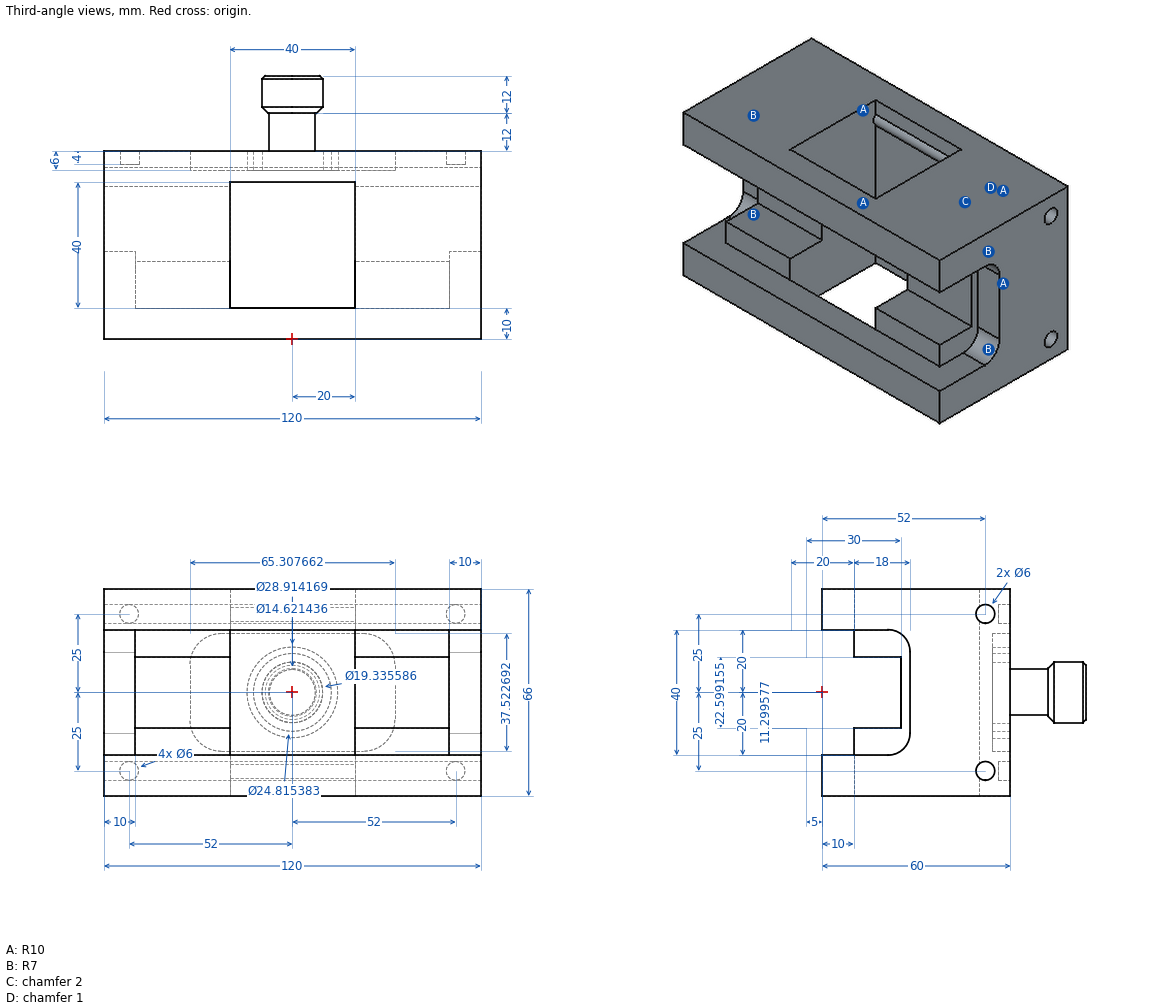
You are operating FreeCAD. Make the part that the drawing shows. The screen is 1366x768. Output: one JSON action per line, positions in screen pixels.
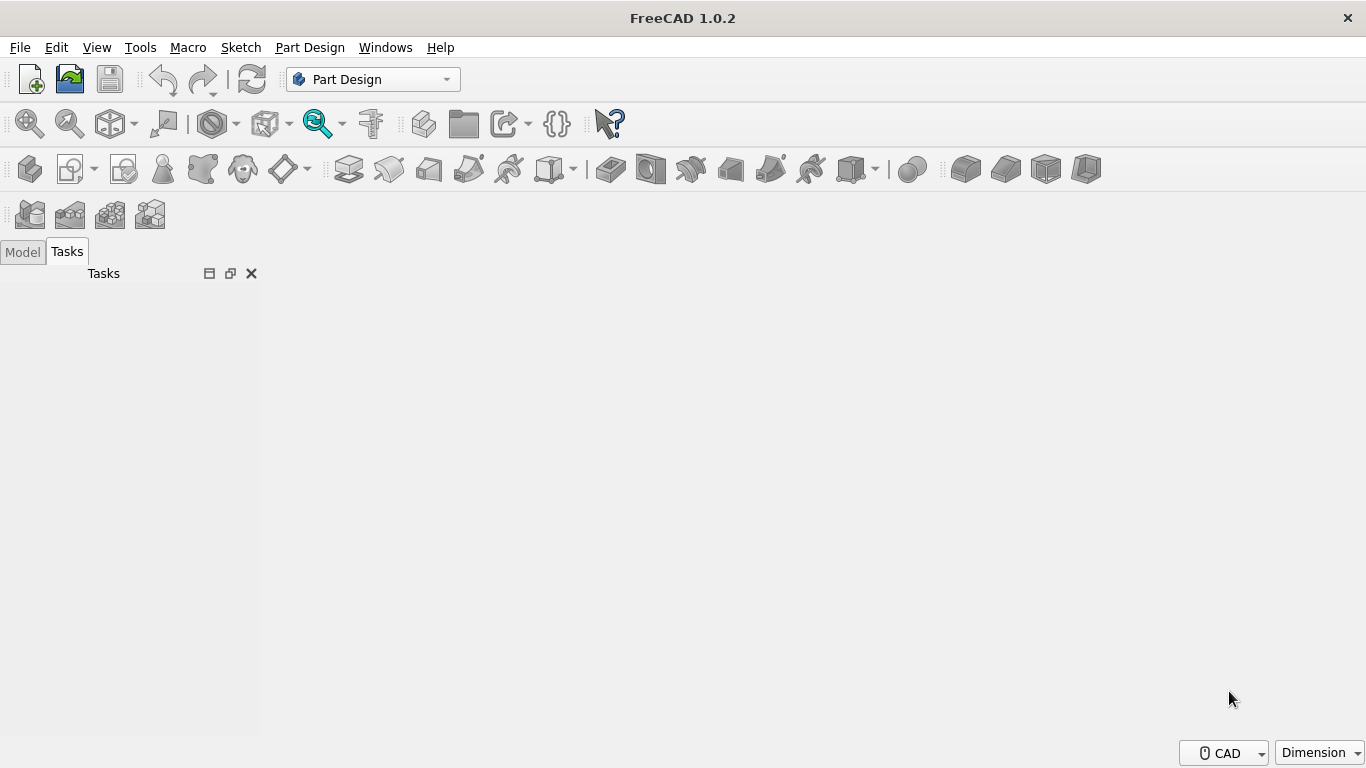
{"action": "left_click", "coordinate": [30, 80]}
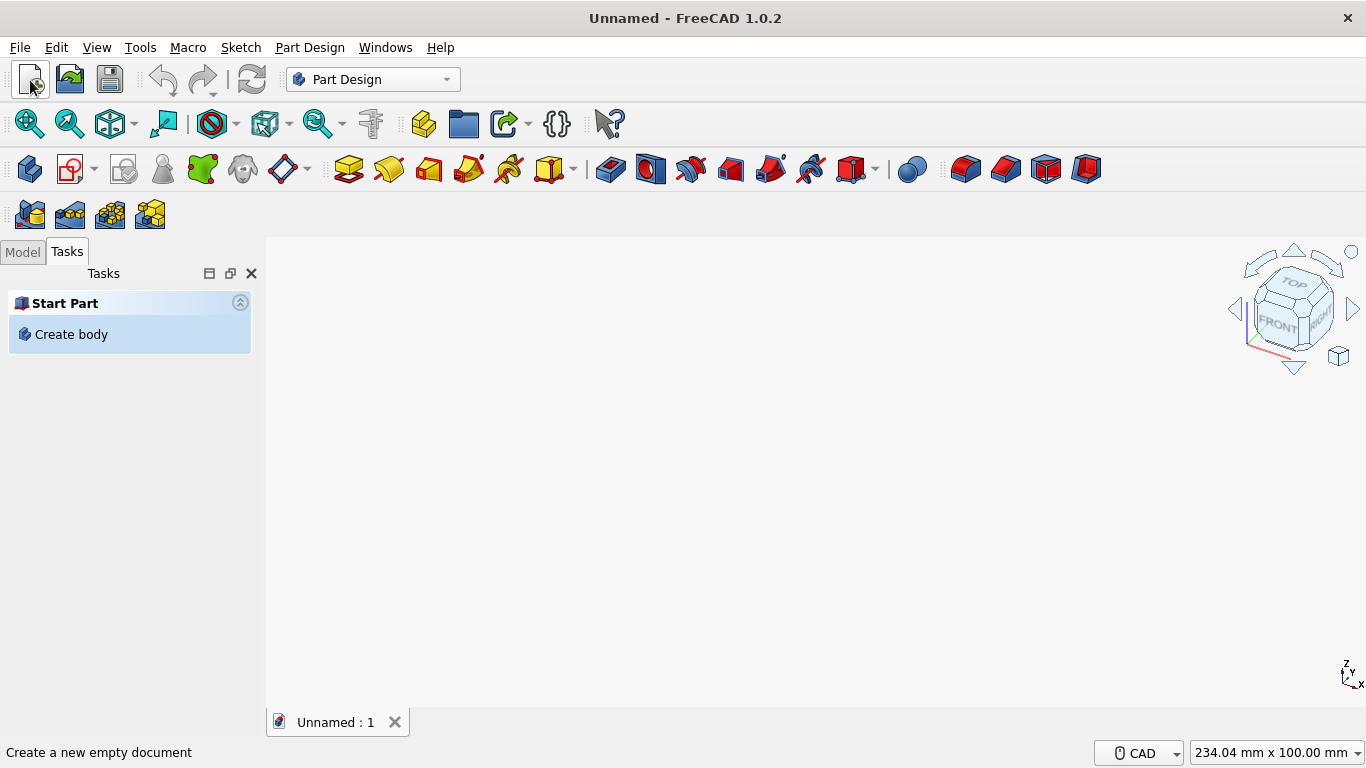
{"action": "left_click", "coordinate": [70, 170]}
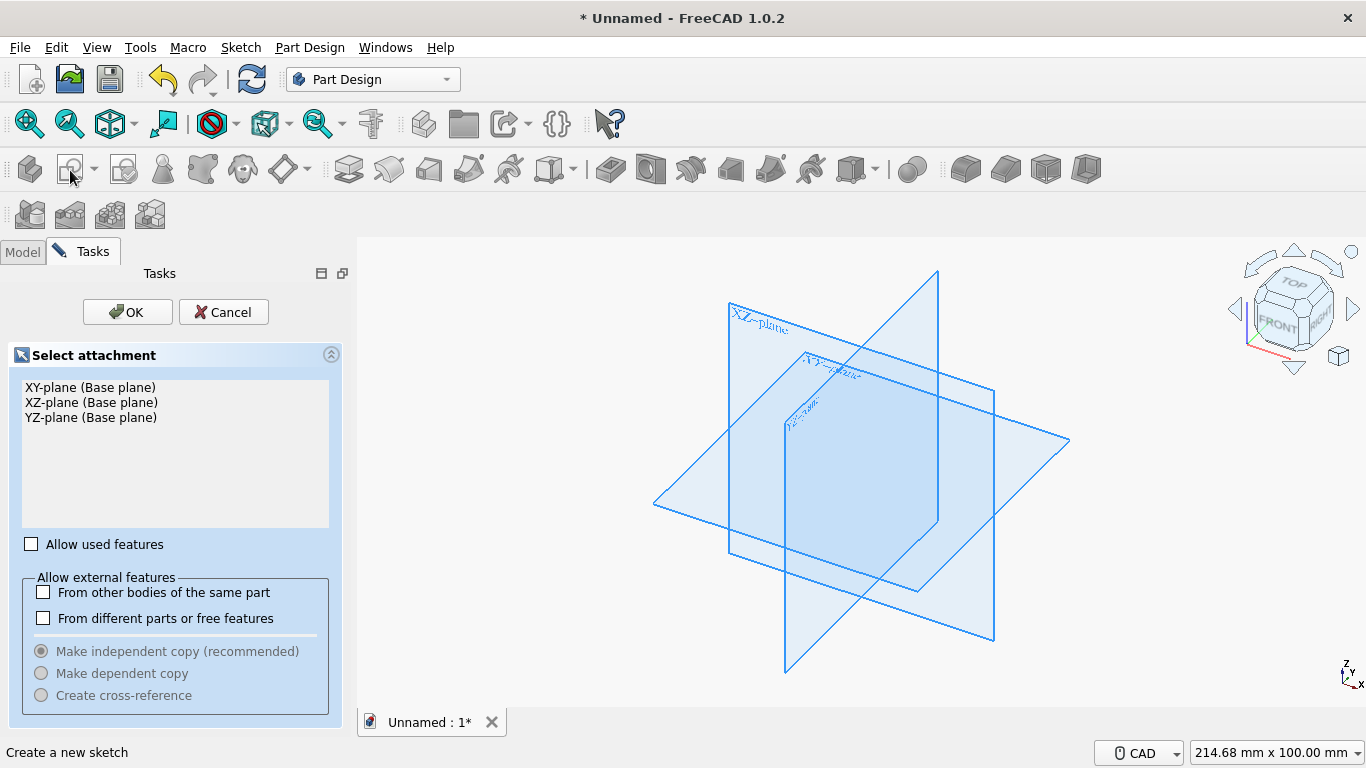
{"action": "left_click", "coordinate": [82, 402]}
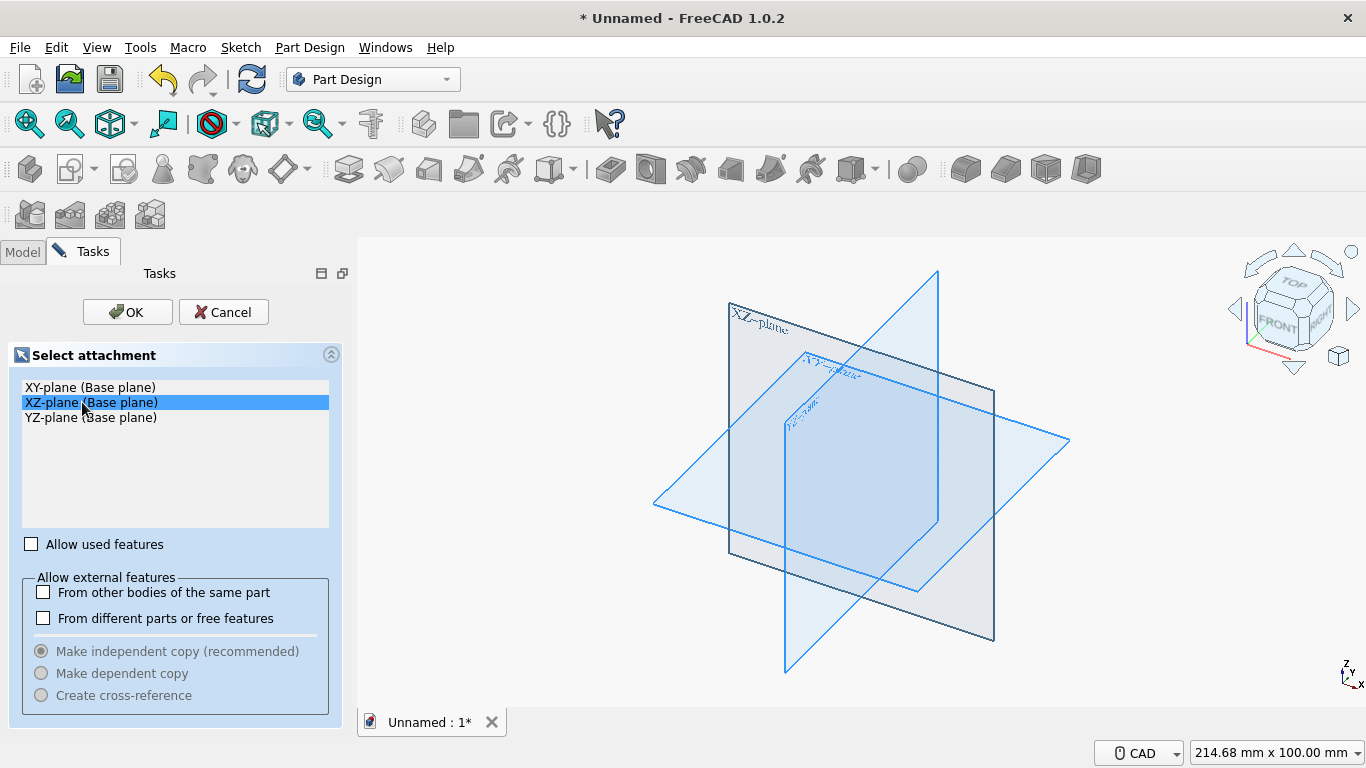
{"action": "left_click", "coordinate": [128, 312]}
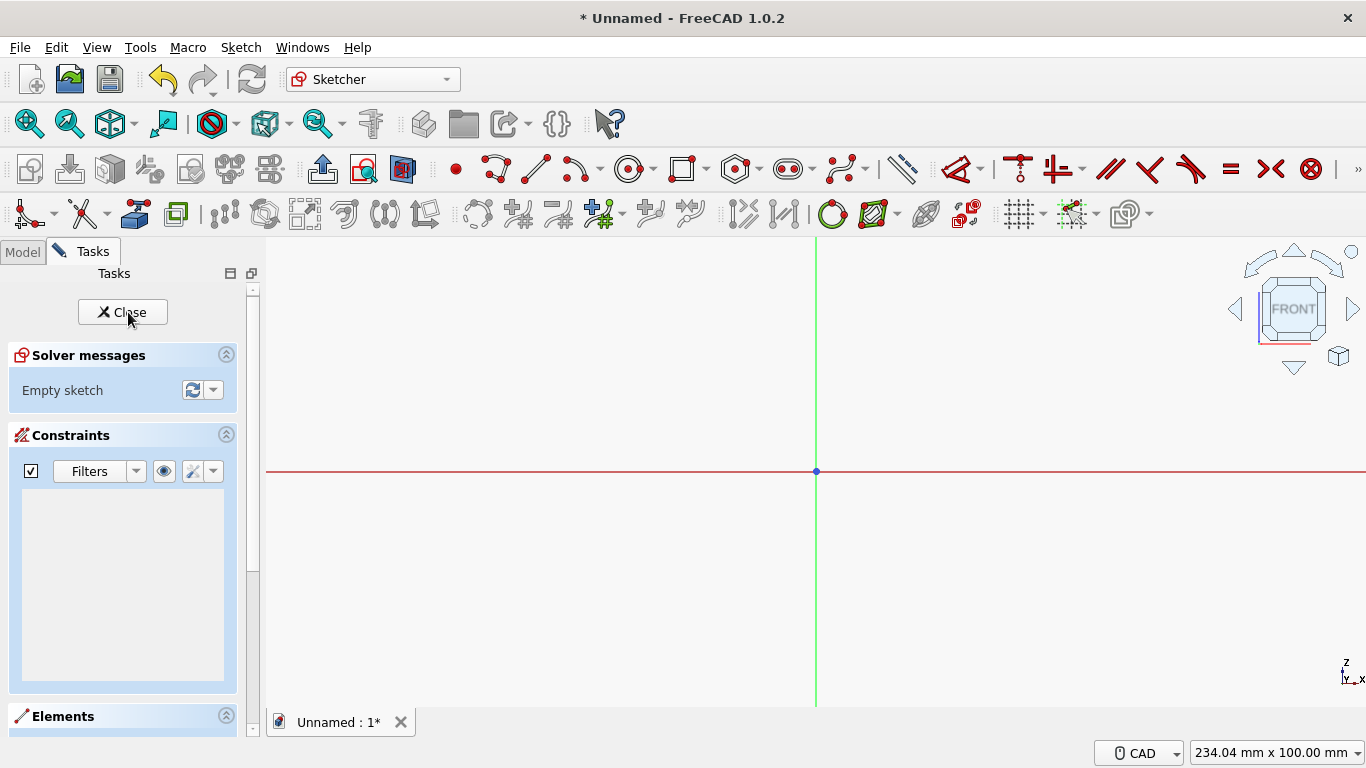
{"action": "left_click", "coordinate": [708, 170]}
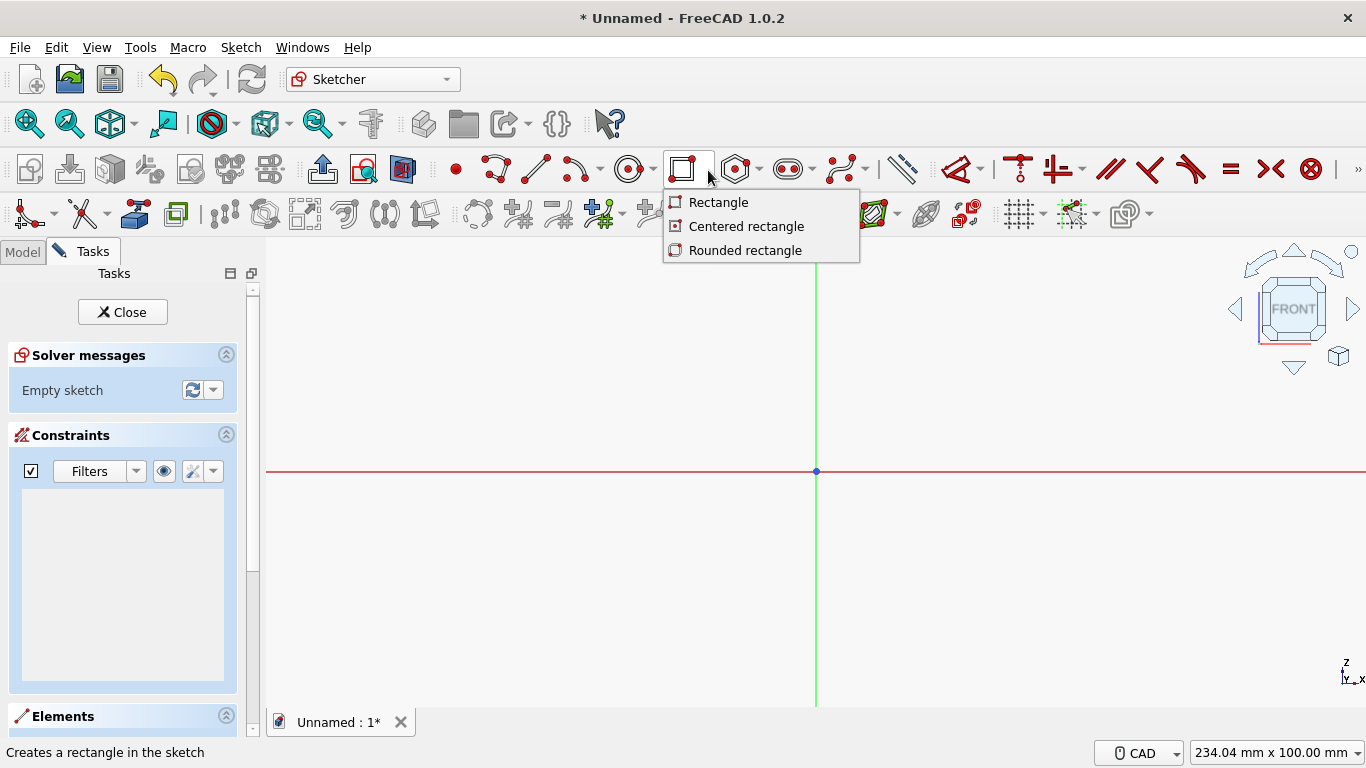
{"action": "left_click", "coordinate": [762, 226]}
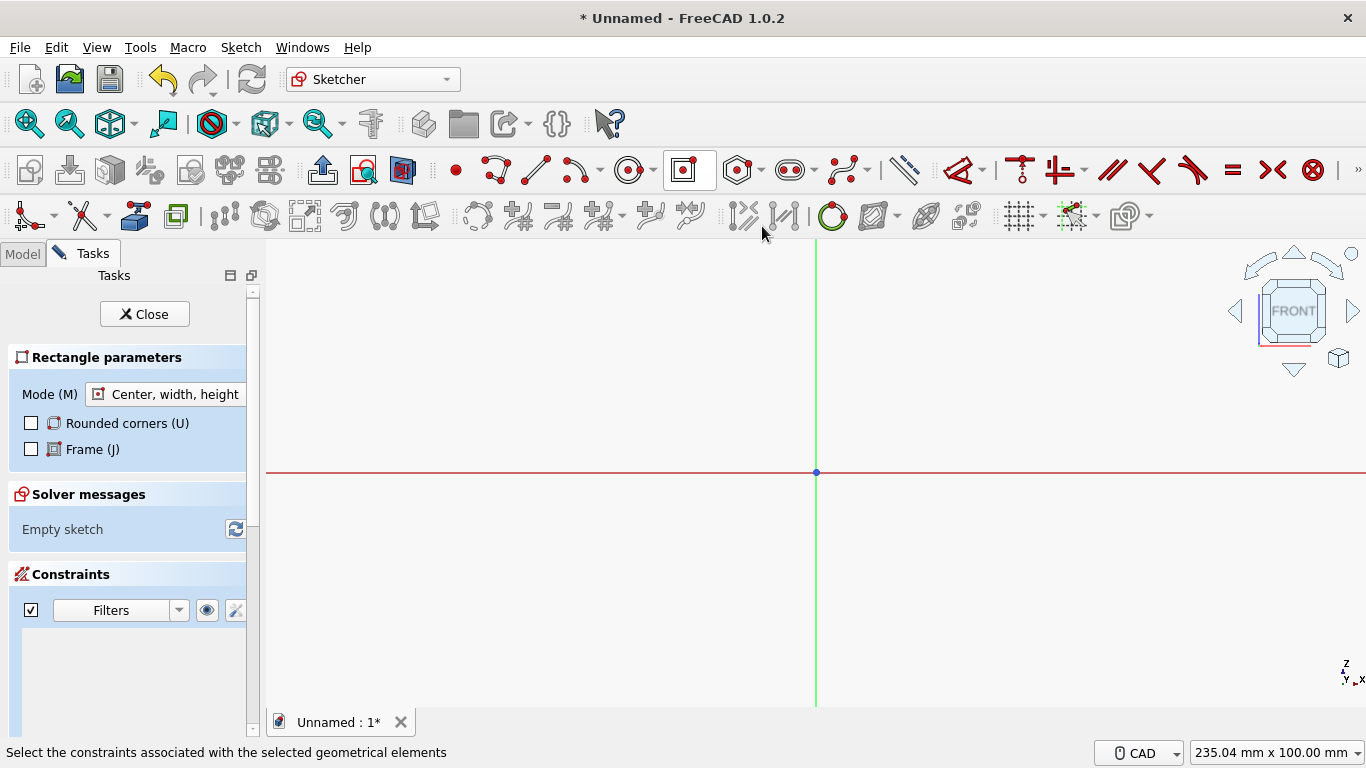
{"action": "left_click", "coordinate": [816, 473]}
{"action": "mouse_move", "coordinate": [1097, 319]}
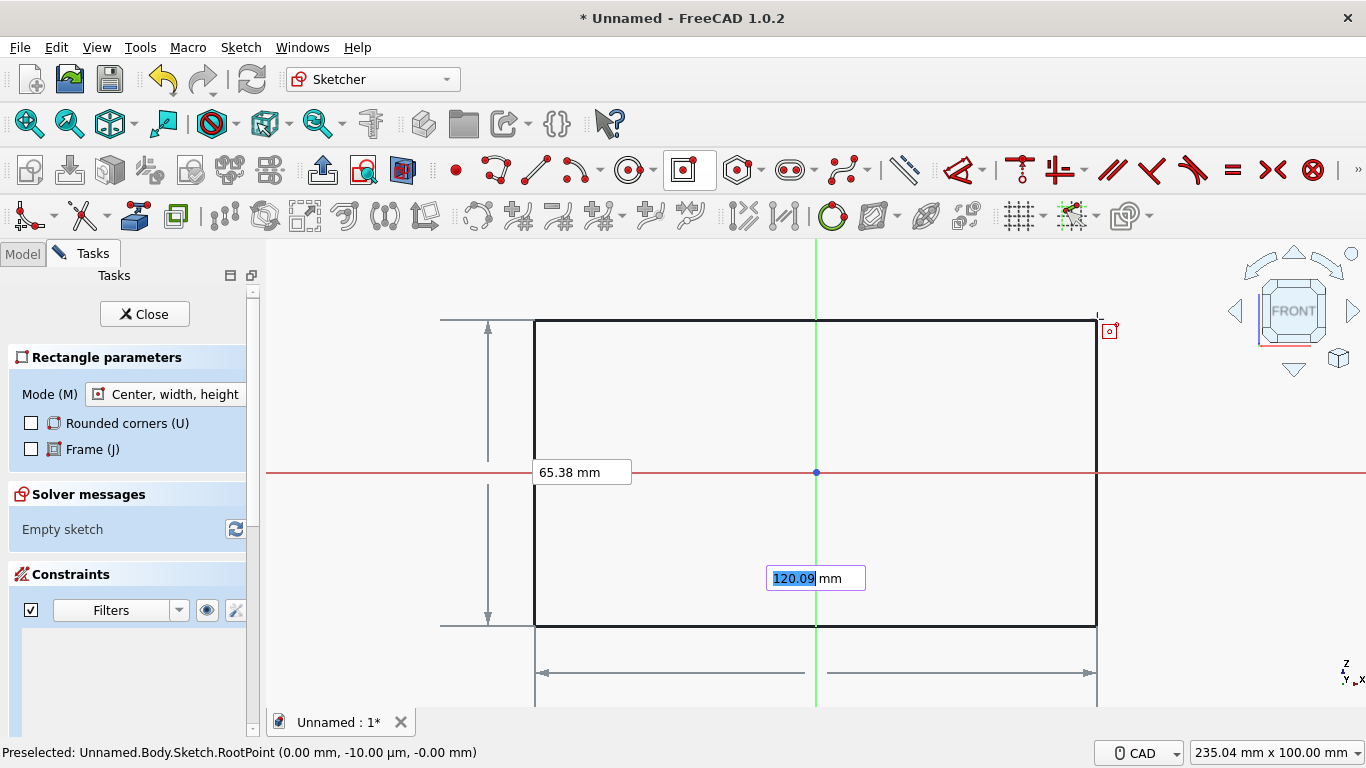
{"action": "type", "text": "120"}
{"action": "key", "text": "Tab"}
{"action": "type", "text": "66"}
{"action": "key", "text": "Return"}
{"action": "key", "text": "Escape"}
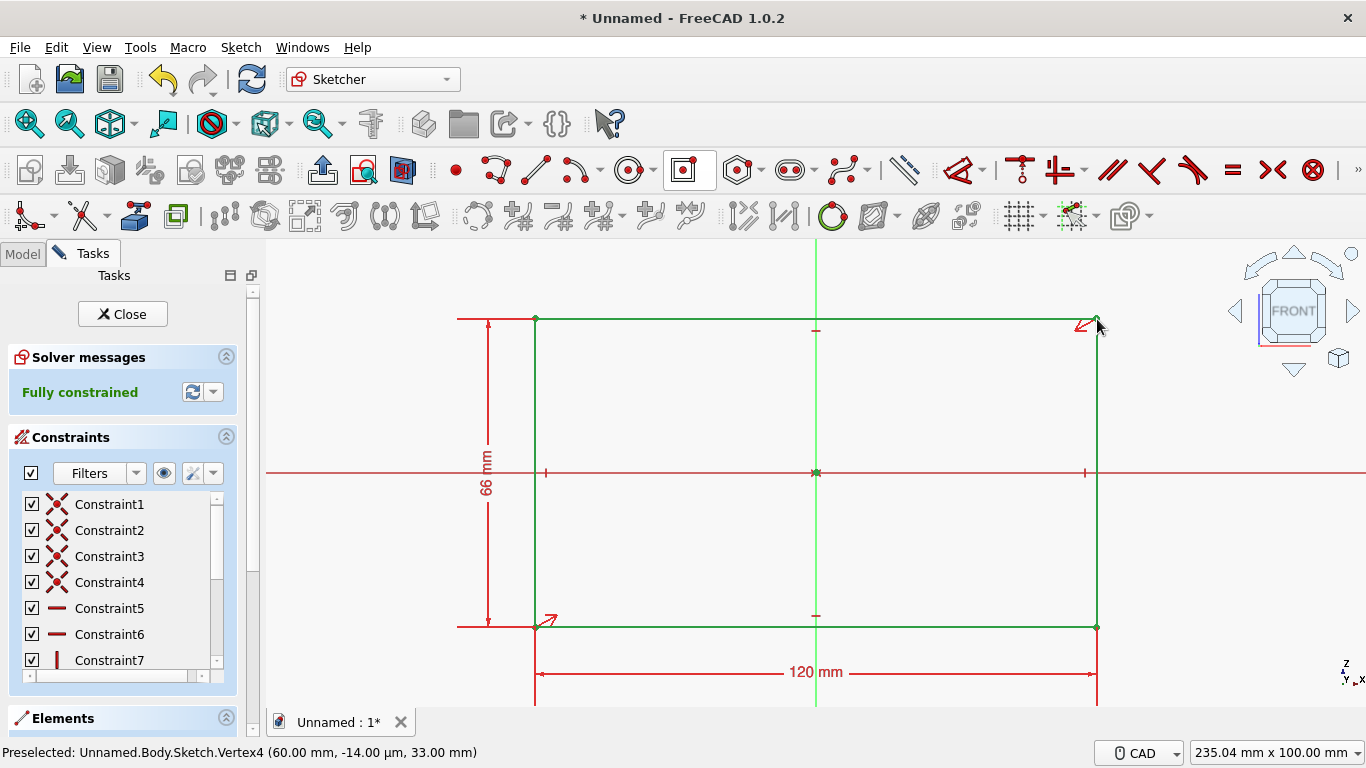
{"action": "left_click", "coordinate": [123, 314]}